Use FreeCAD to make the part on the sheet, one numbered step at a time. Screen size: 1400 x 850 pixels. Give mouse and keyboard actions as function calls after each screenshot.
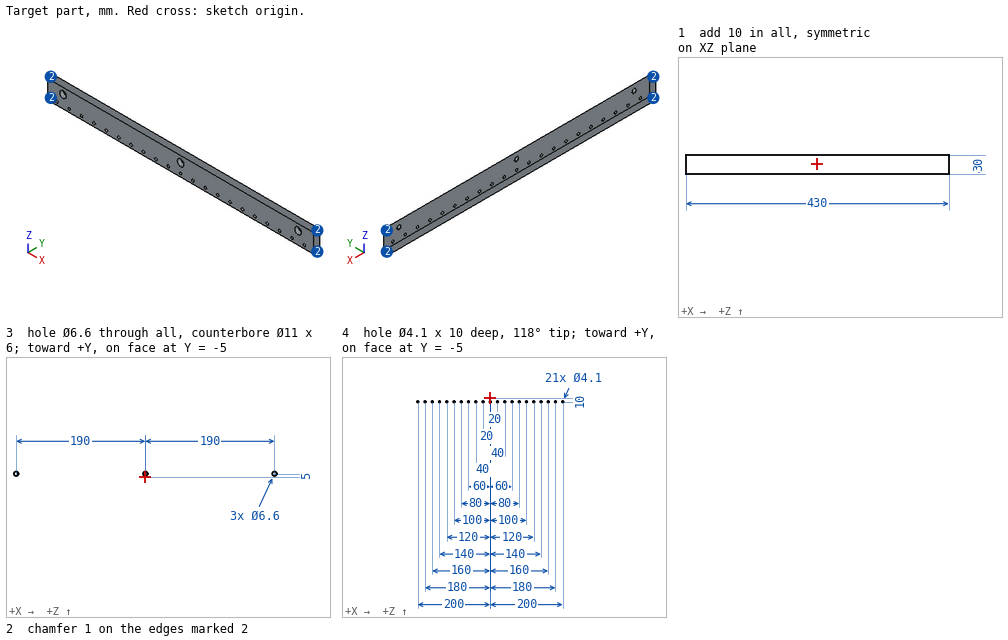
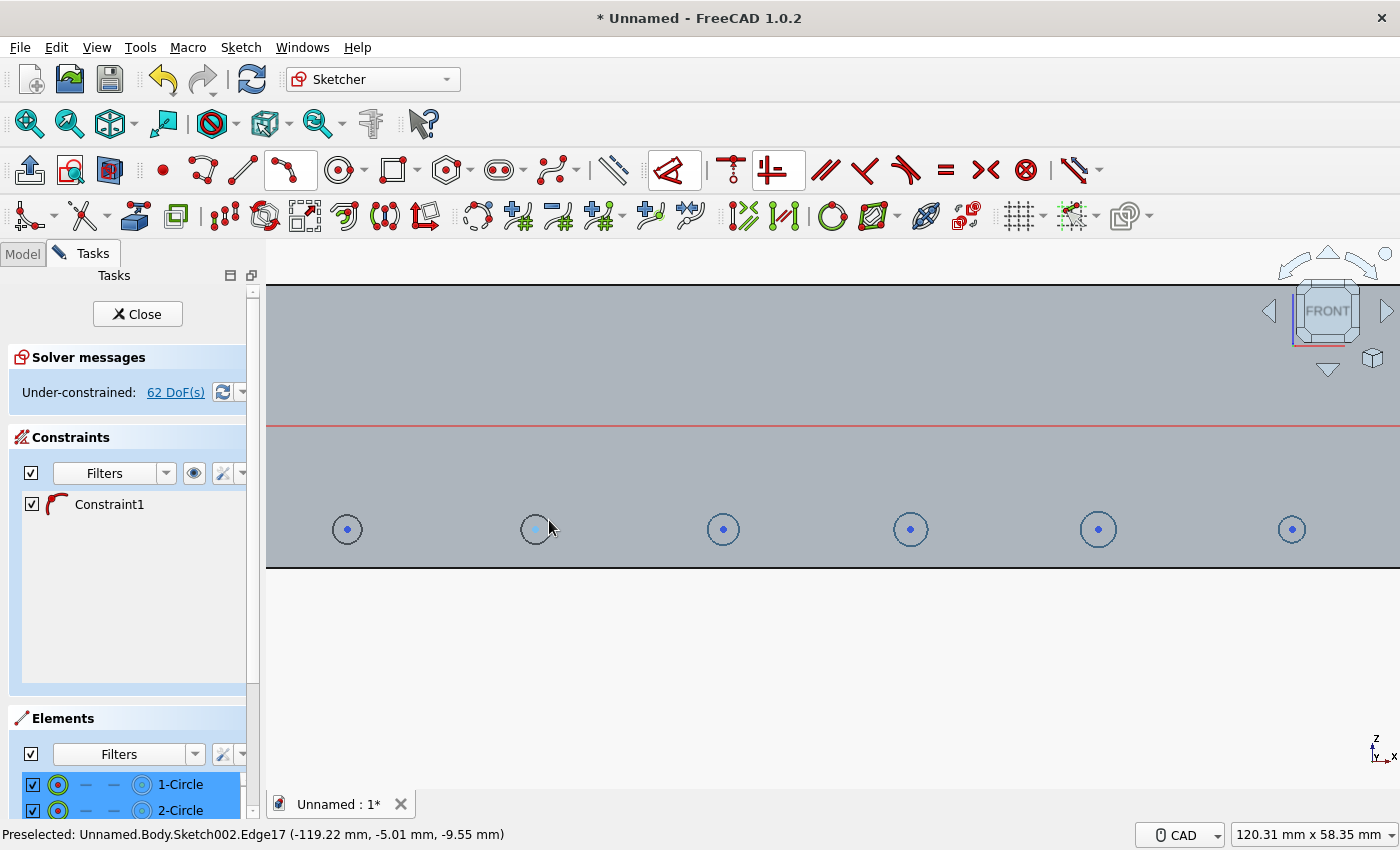
click(546, 519)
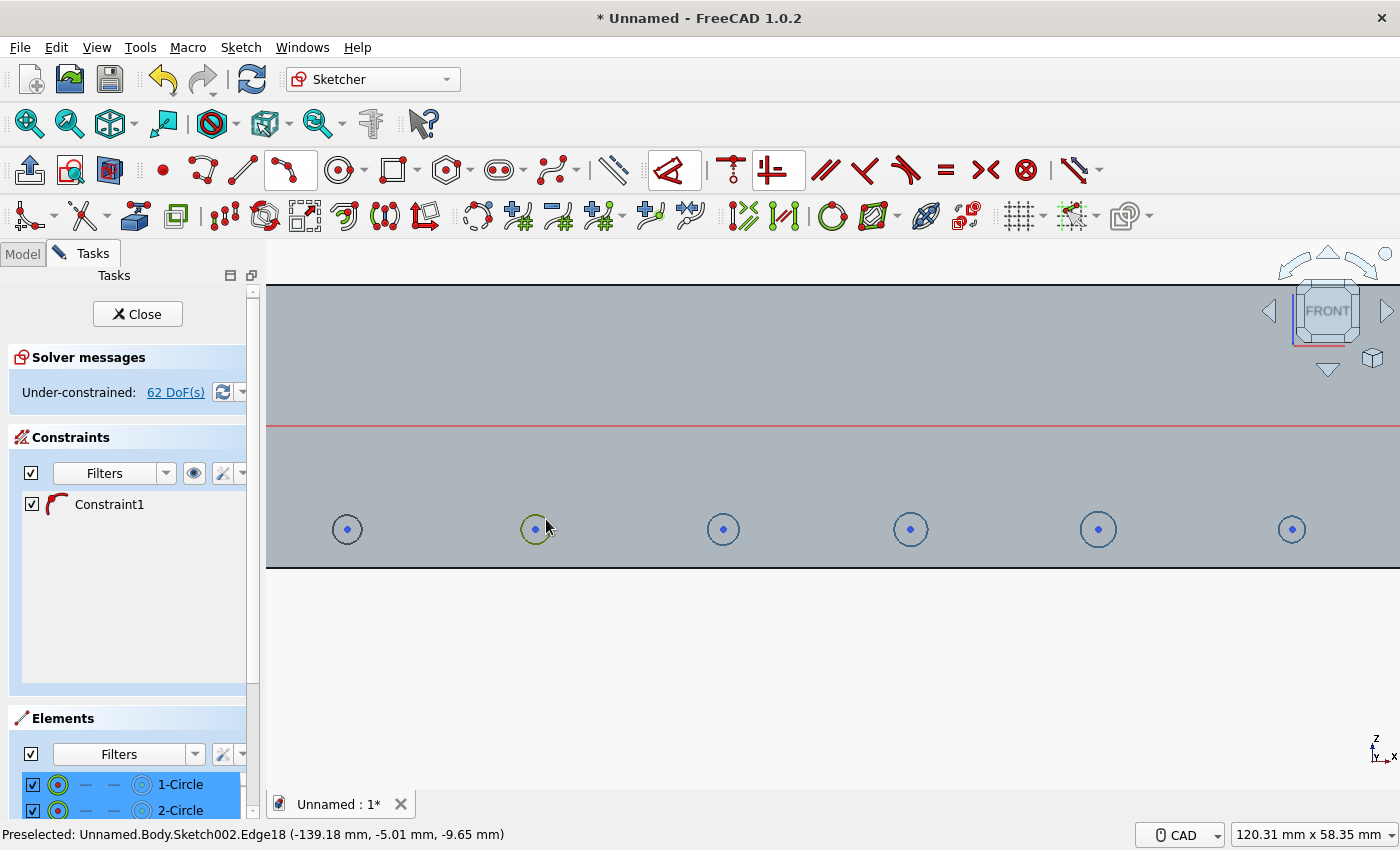
click(357, 519)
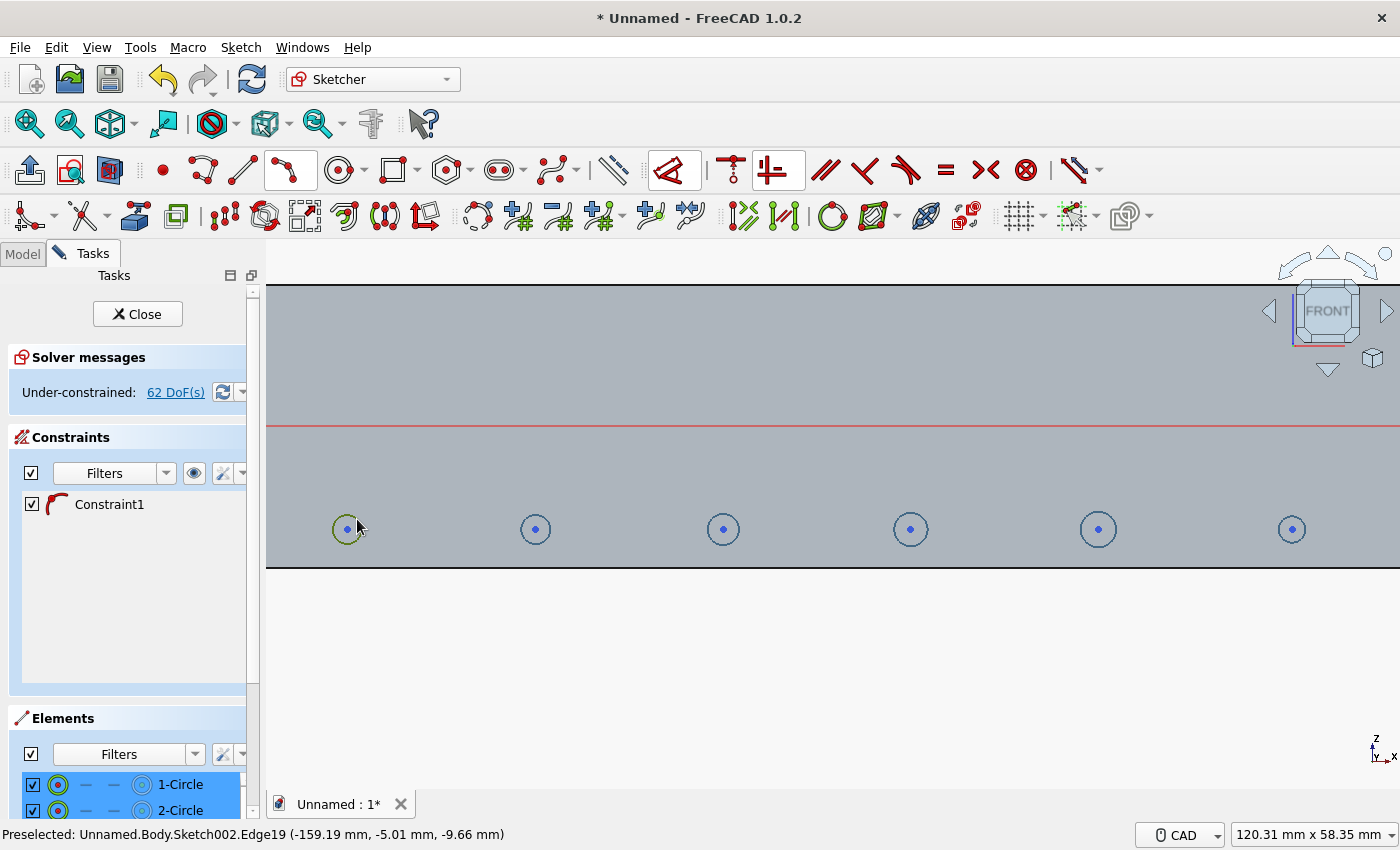
scroll(548, 520, down, 9)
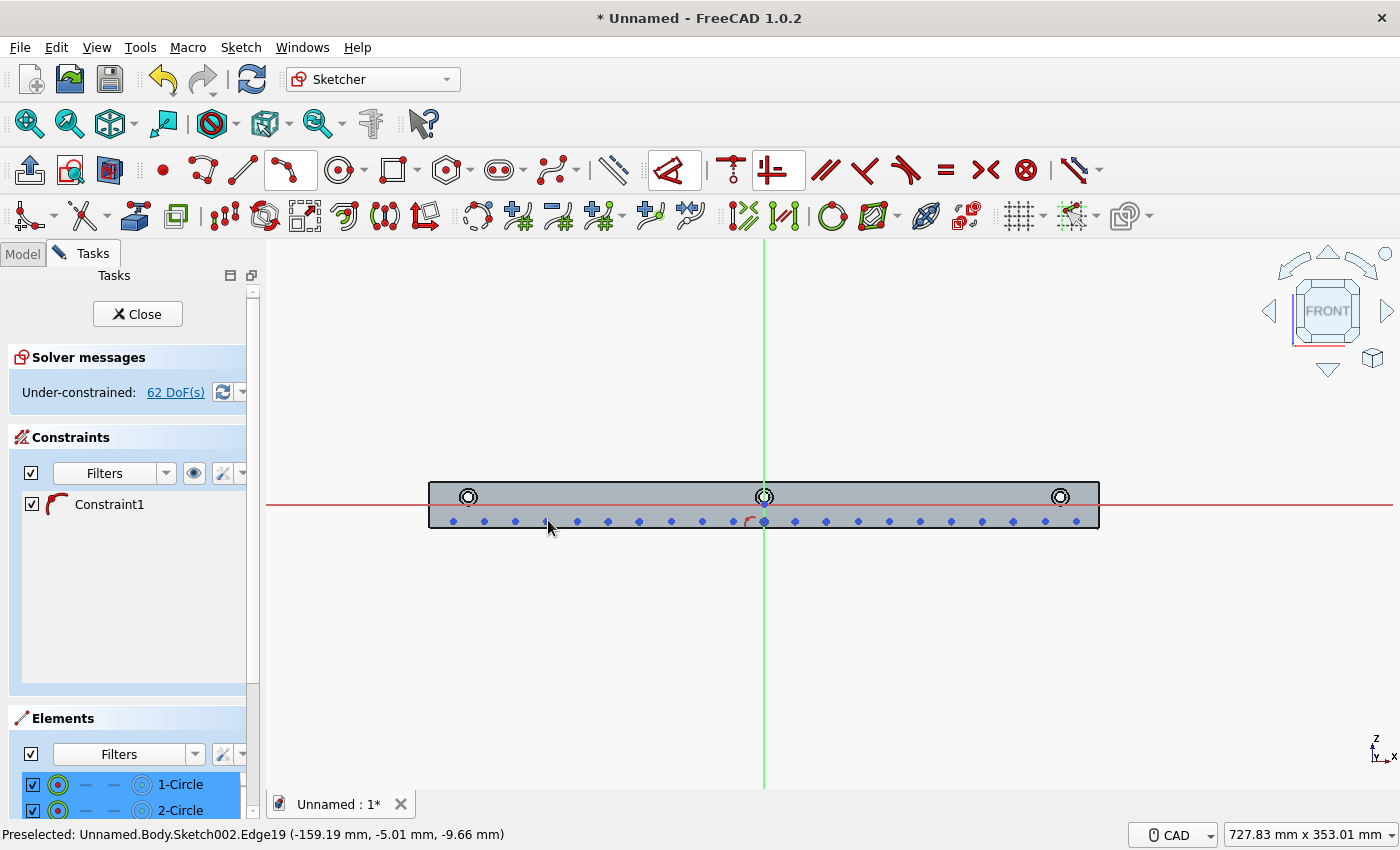
scroll(486, 520, up, 9)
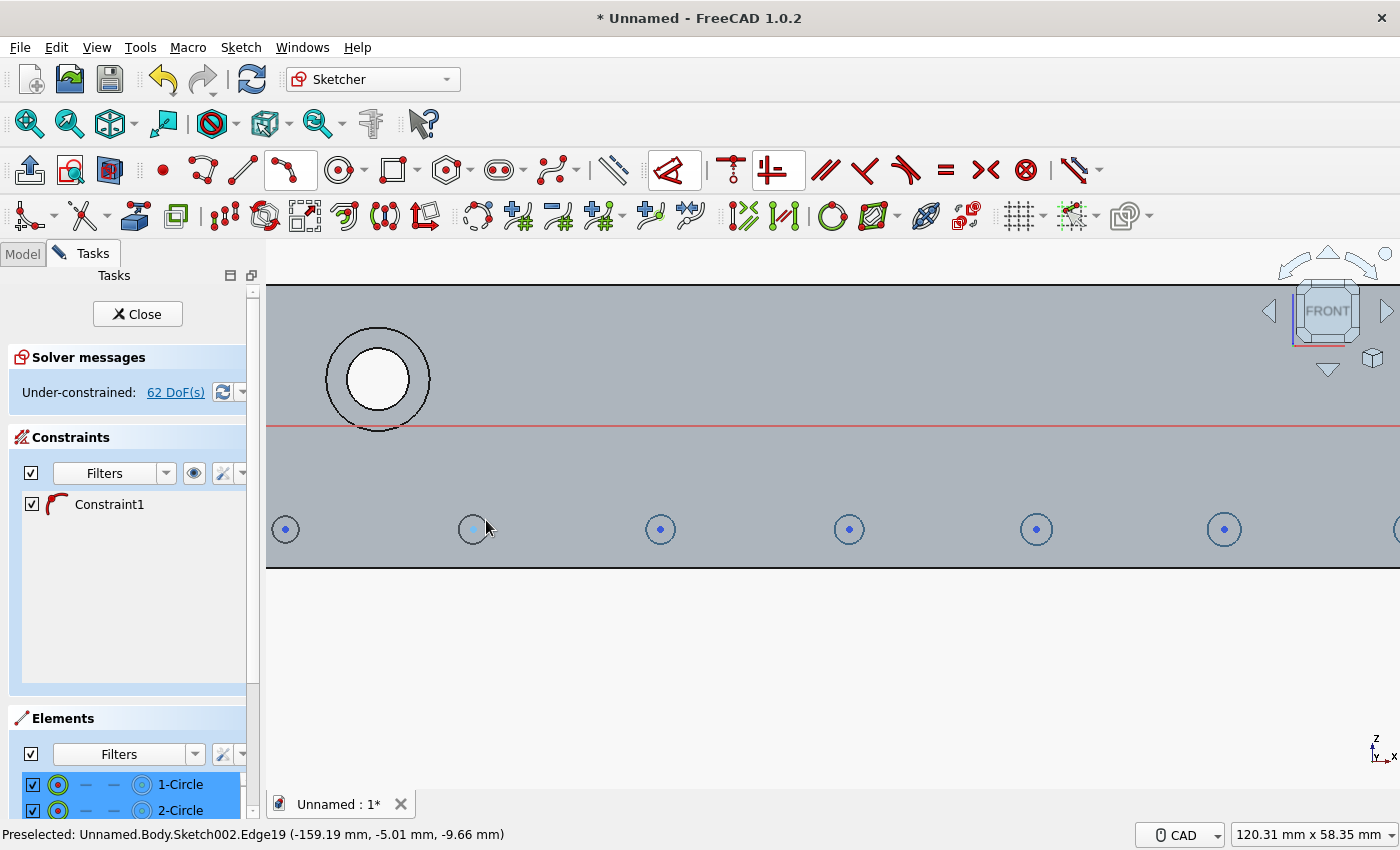
click(483, 519)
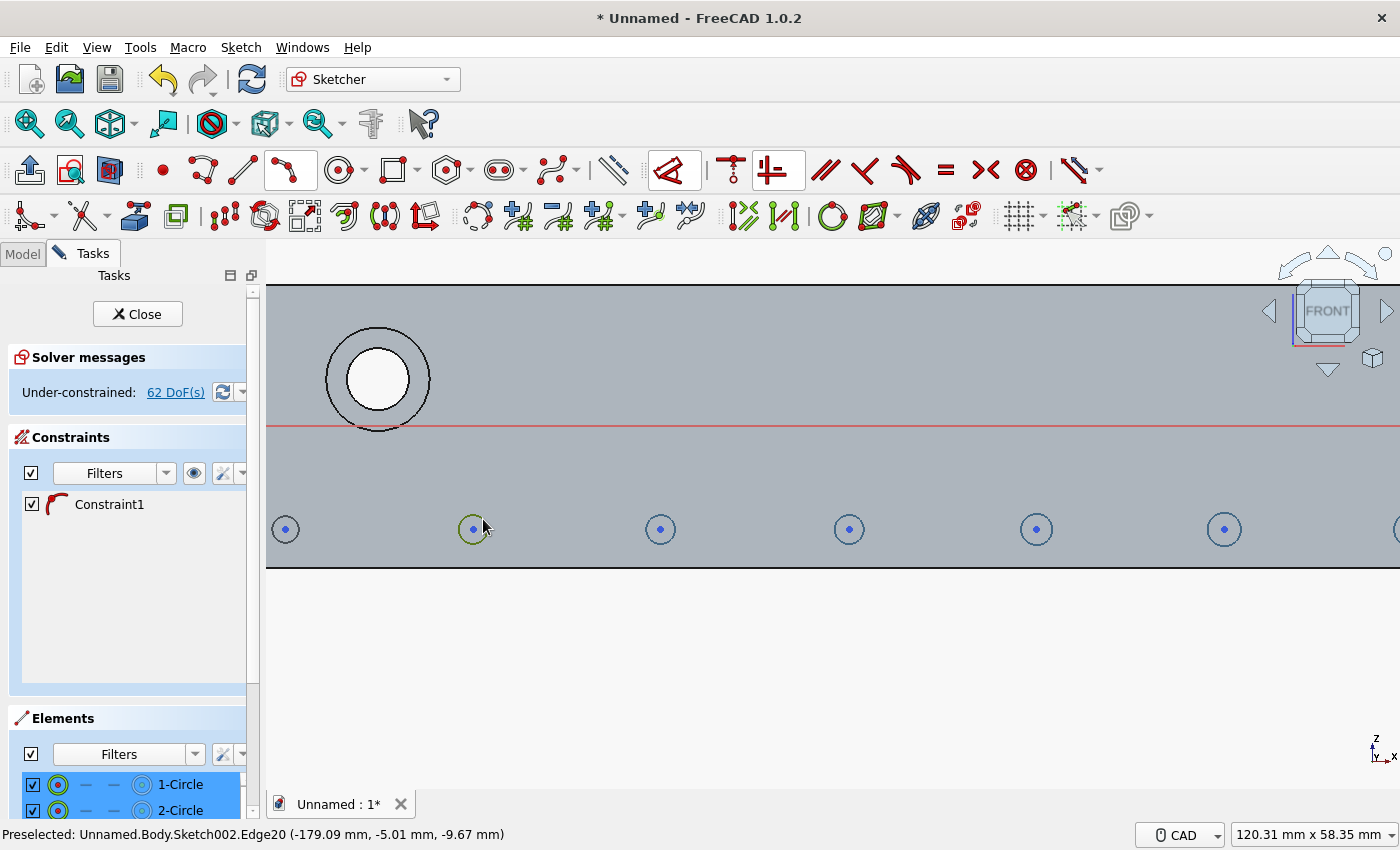
click(295, 520)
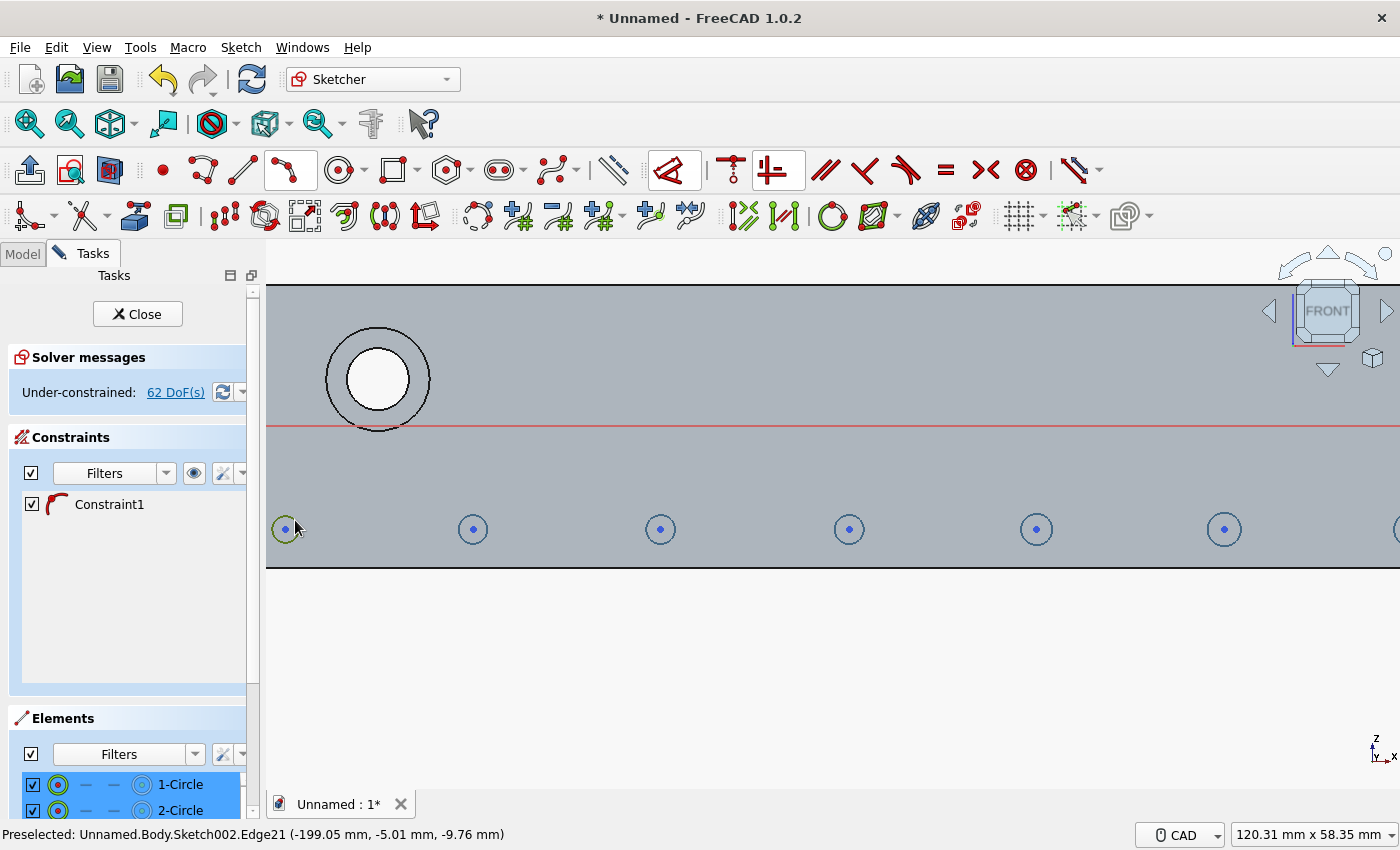
click(946, 170)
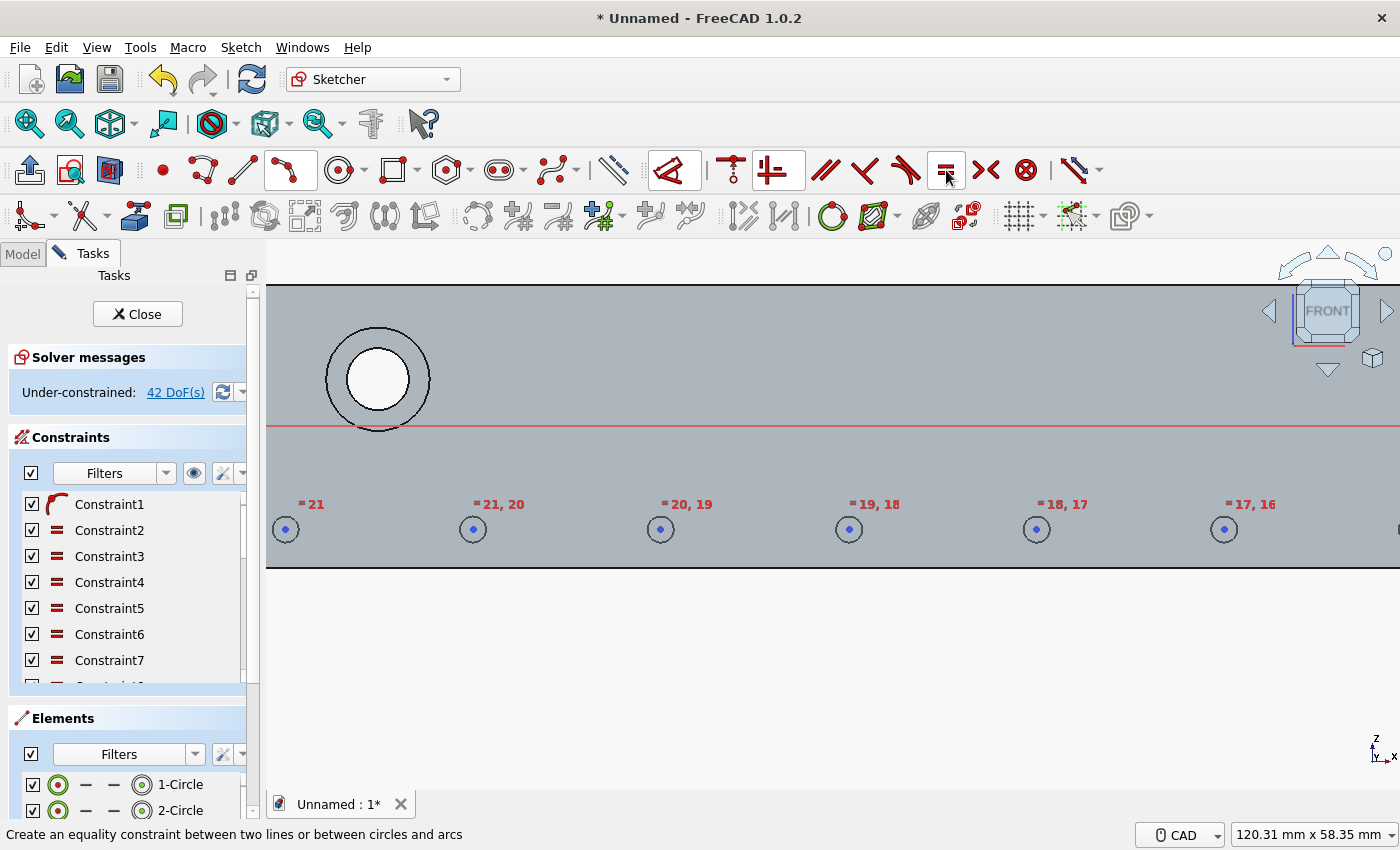
scroll(486, 520, down, 9)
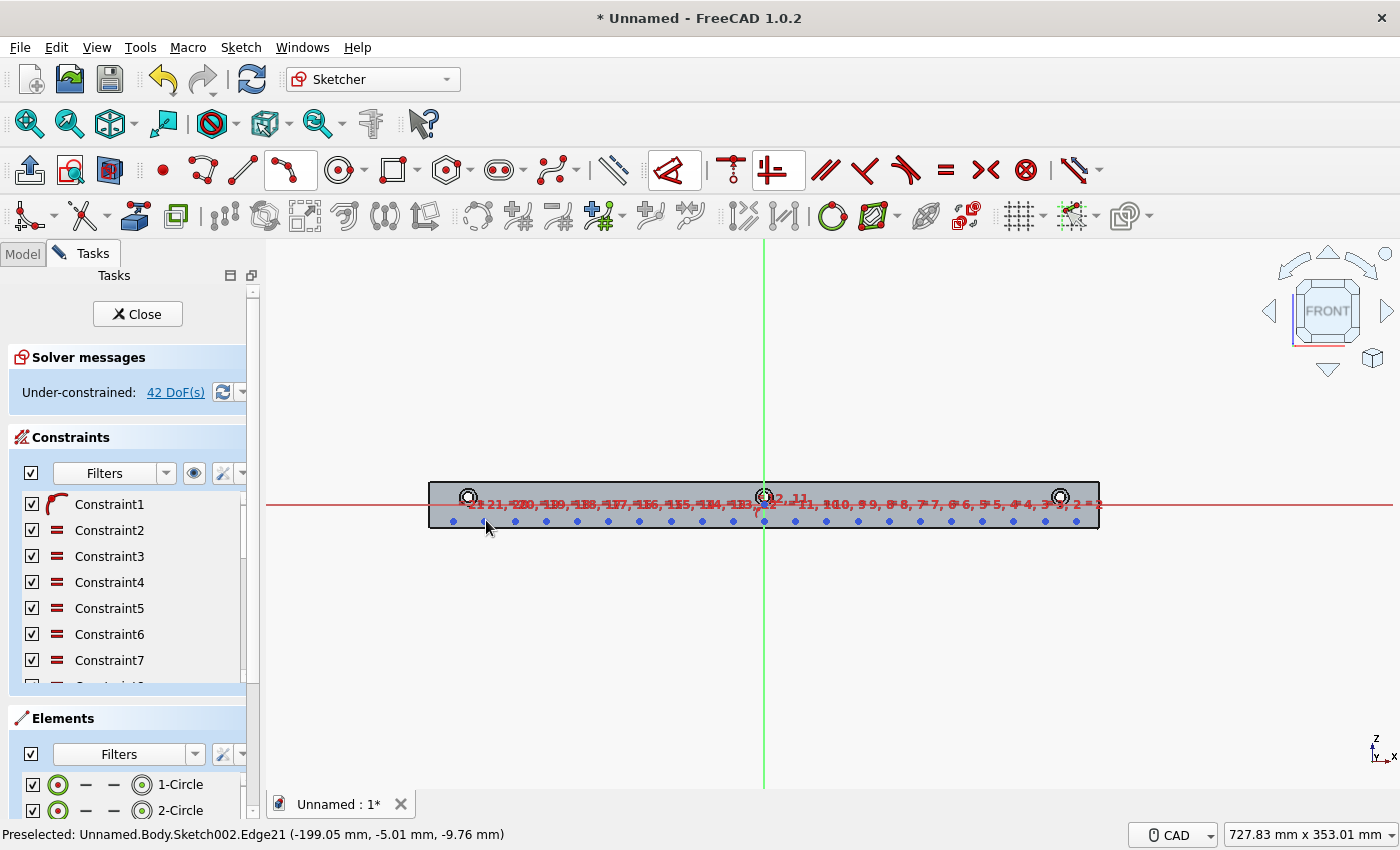
click(1076, 522)